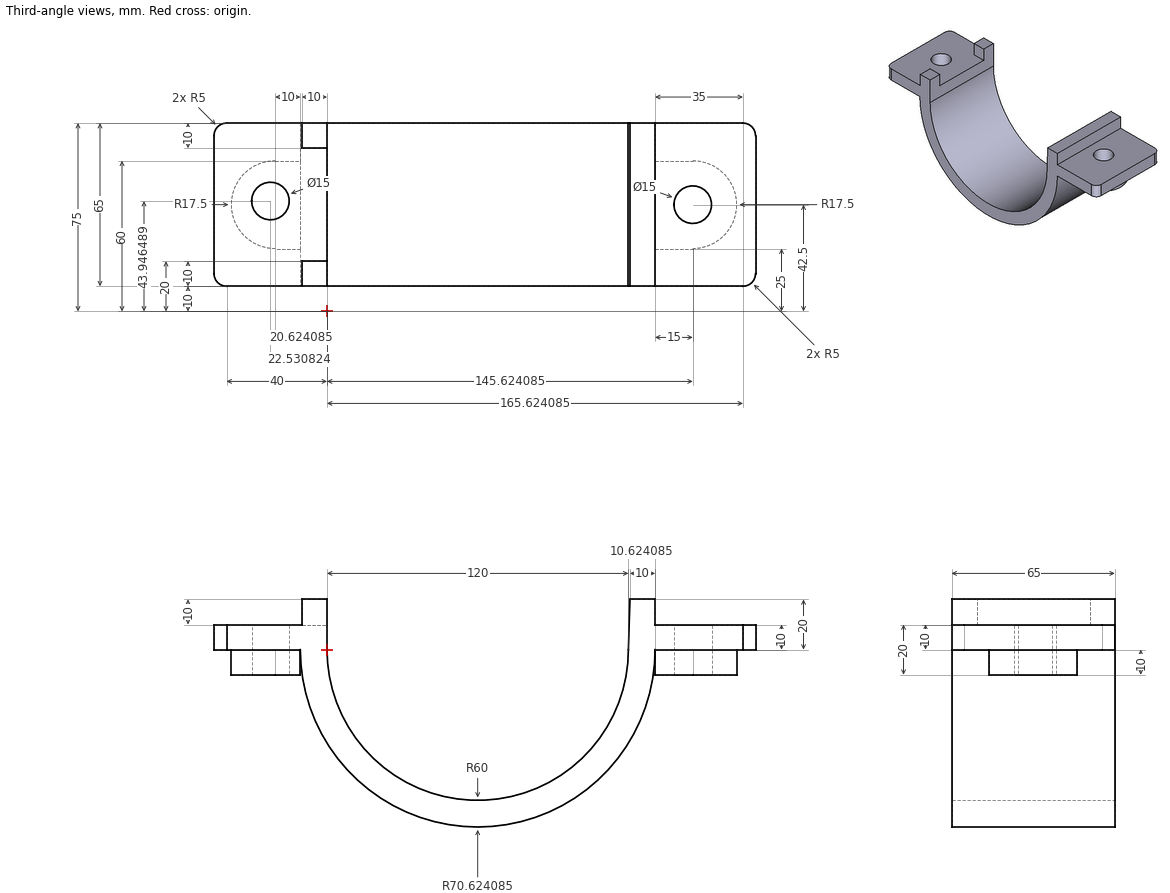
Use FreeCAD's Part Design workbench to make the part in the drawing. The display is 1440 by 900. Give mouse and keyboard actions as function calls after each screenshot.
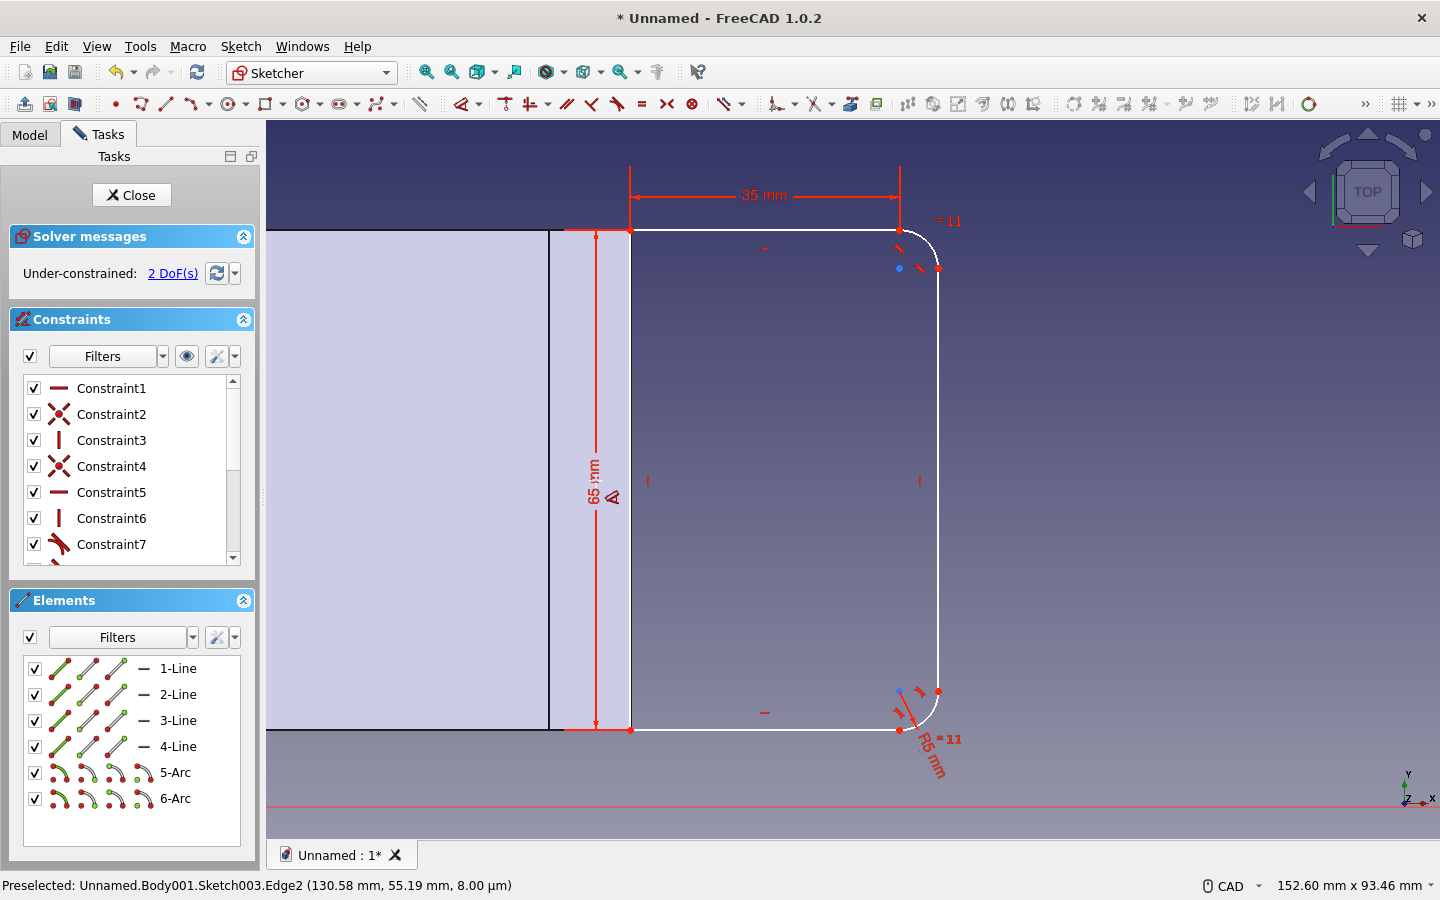
click(900, 230)
click(958, 518)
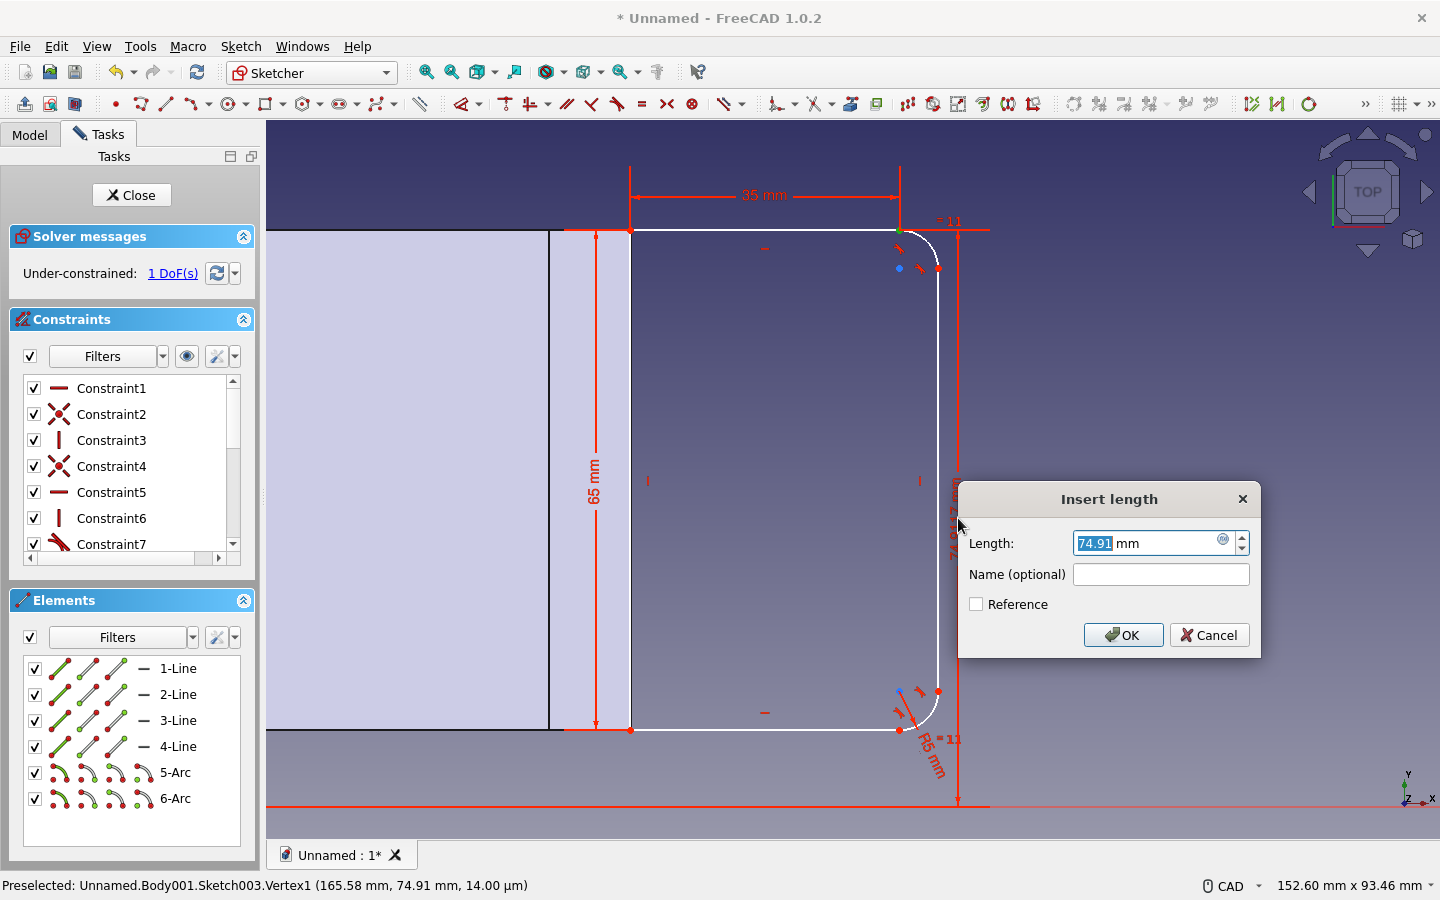
text(75)
key(Return)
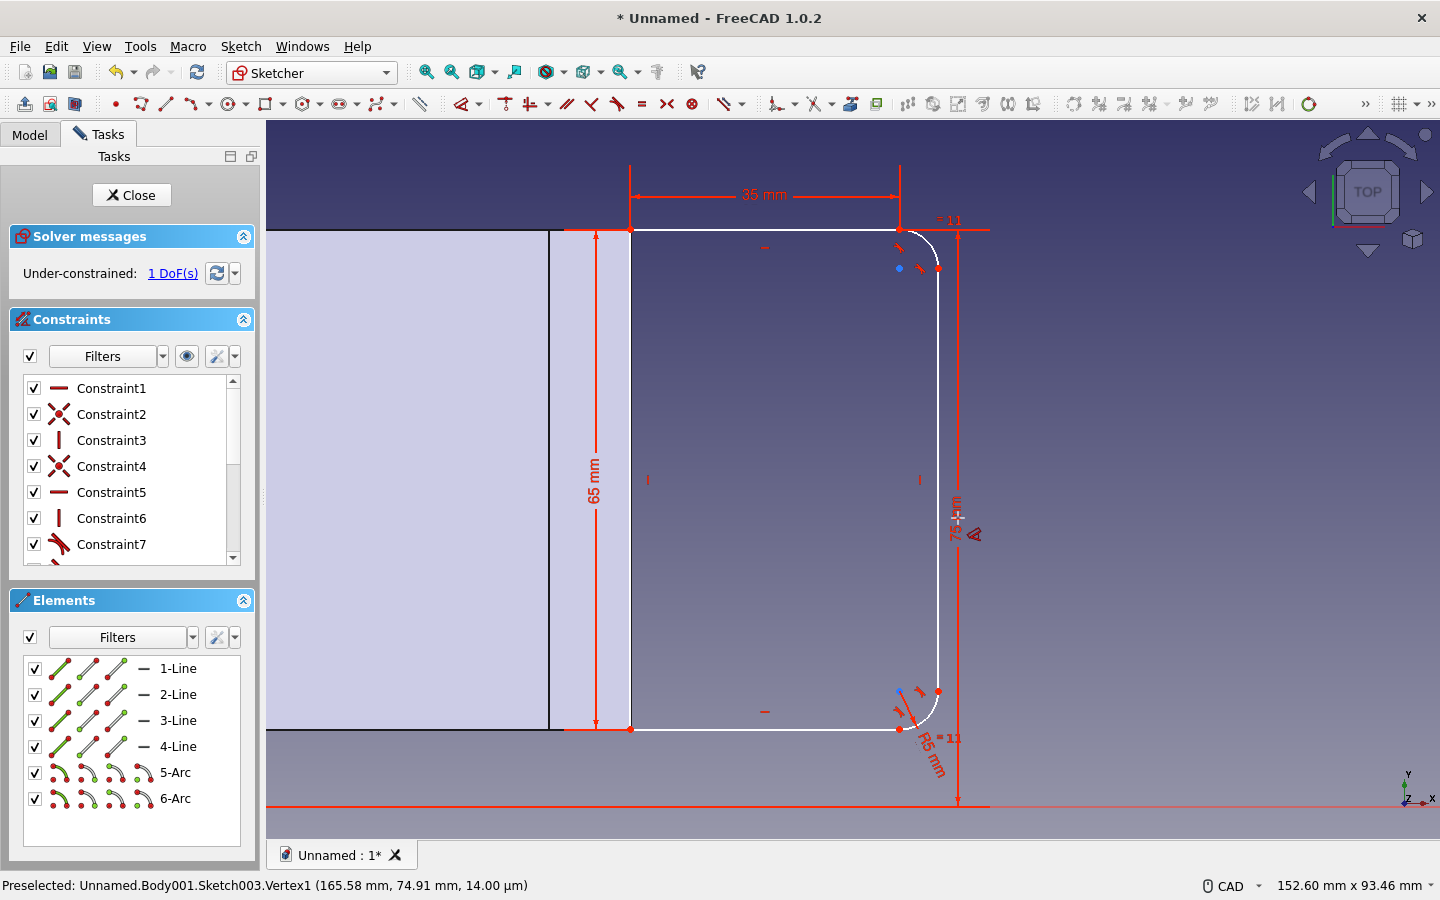
click(900, 230)
click(597, 196)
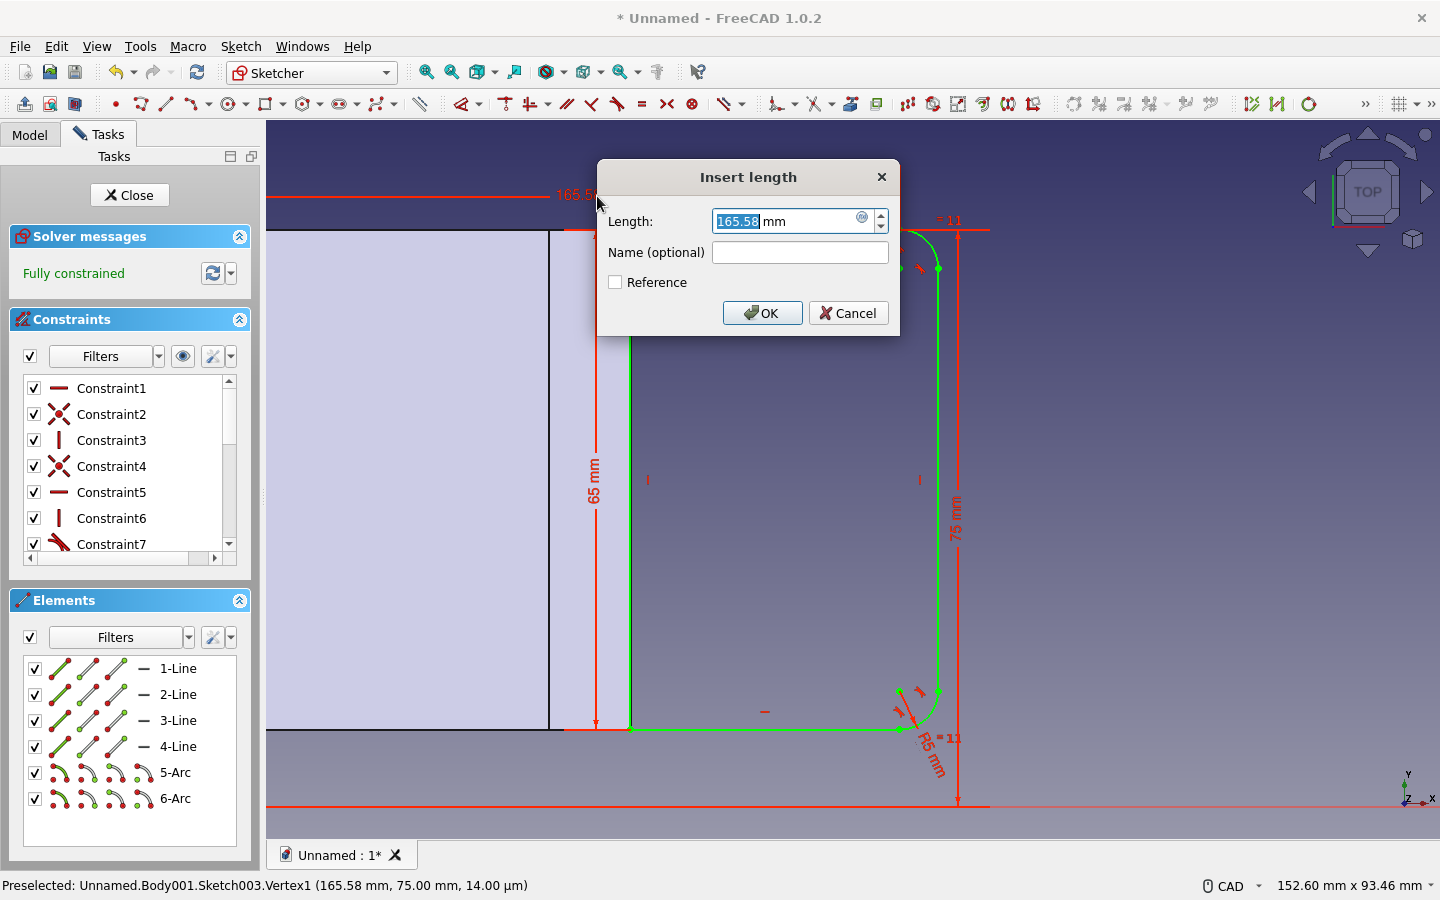
text(165.624085)
key(Return)
key(Escape)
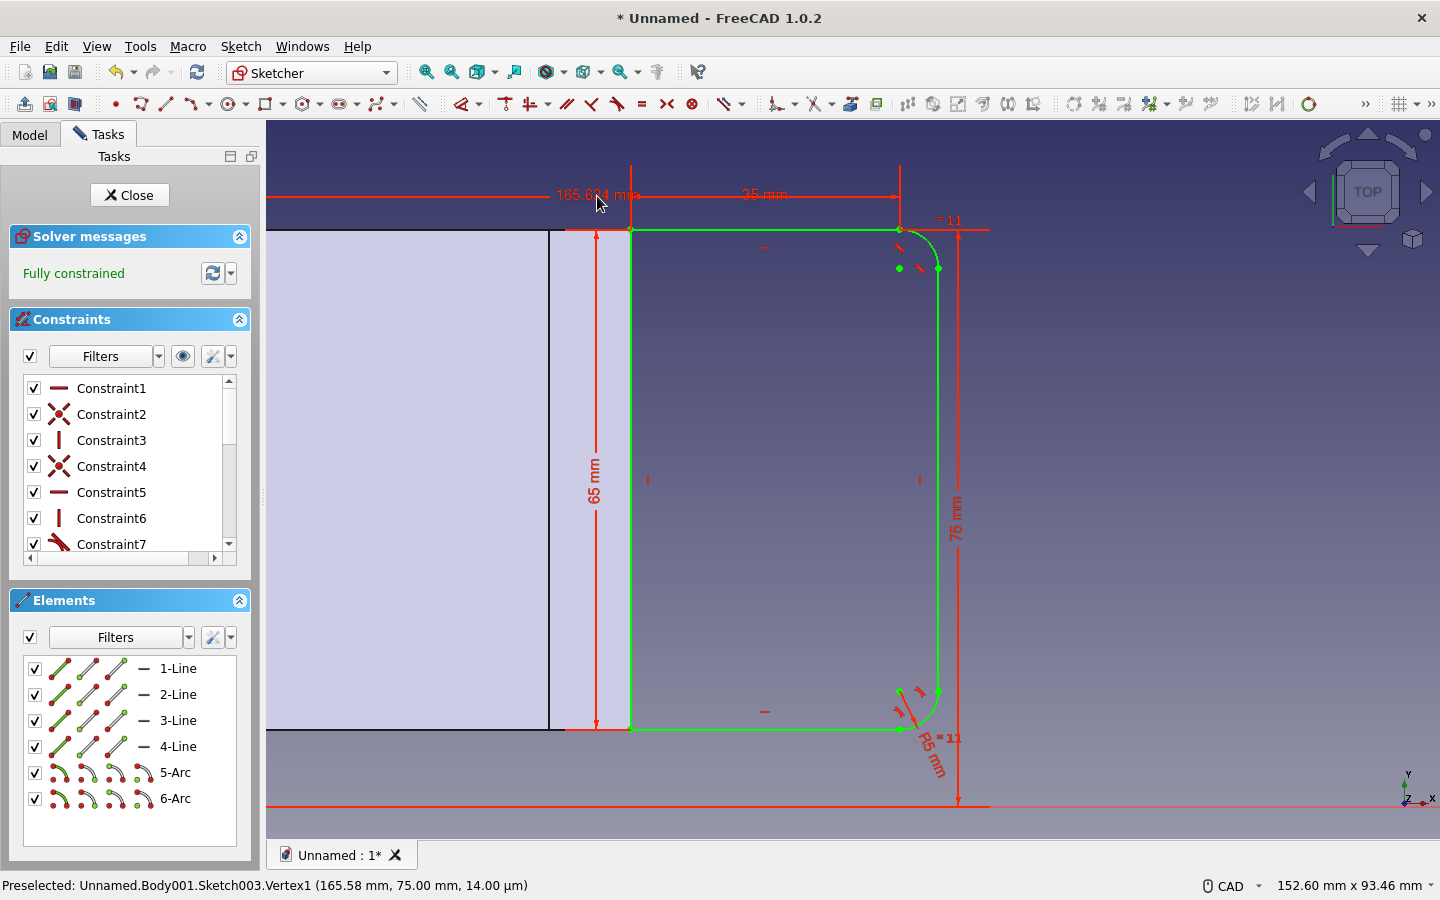
click(130, 195)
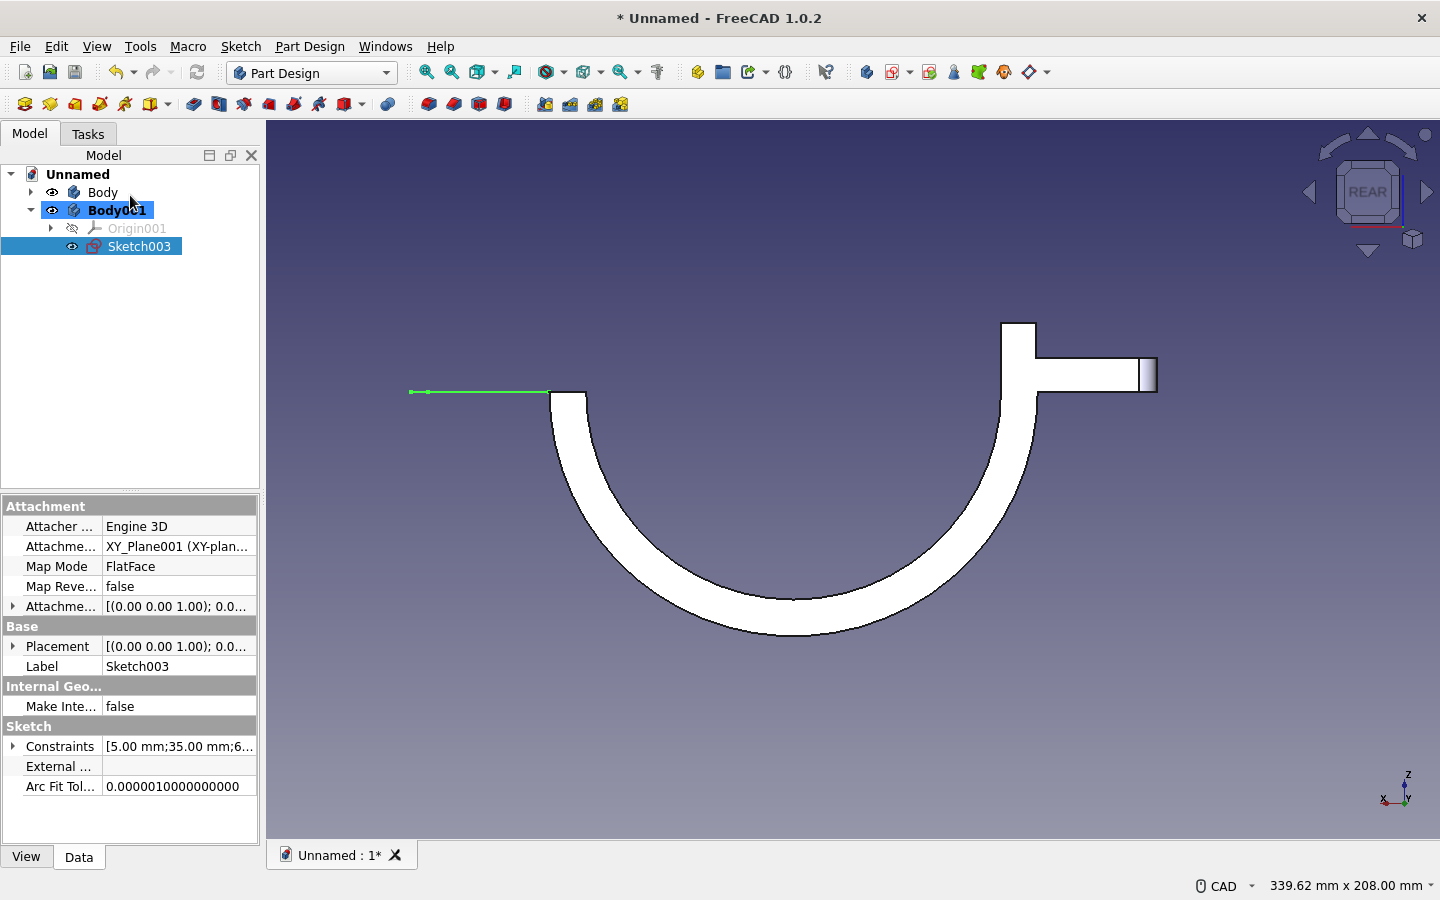
click(25, 104)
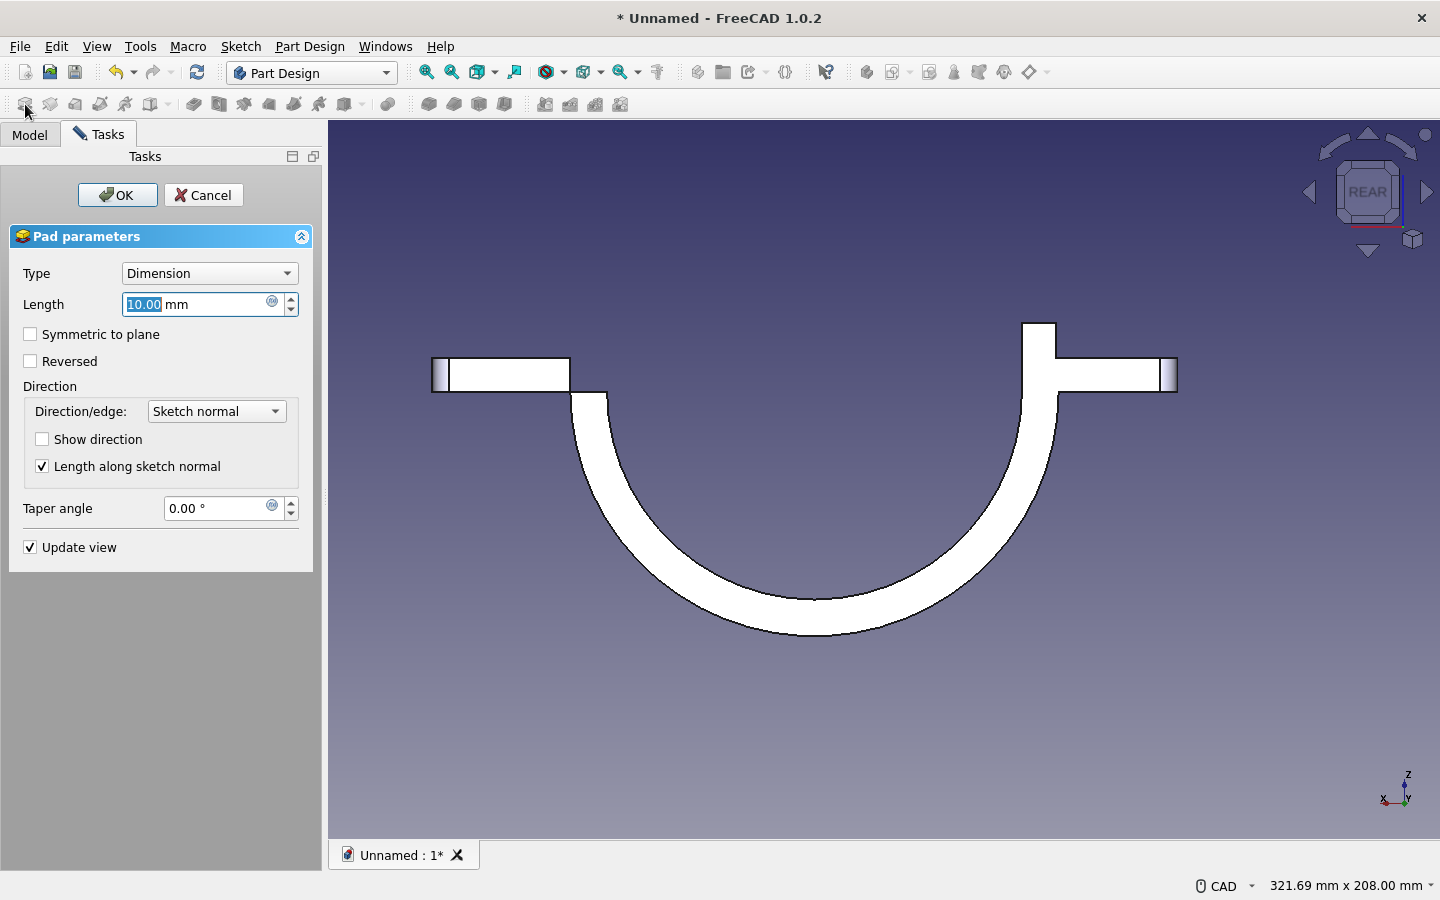
text(10)
key(Tab)